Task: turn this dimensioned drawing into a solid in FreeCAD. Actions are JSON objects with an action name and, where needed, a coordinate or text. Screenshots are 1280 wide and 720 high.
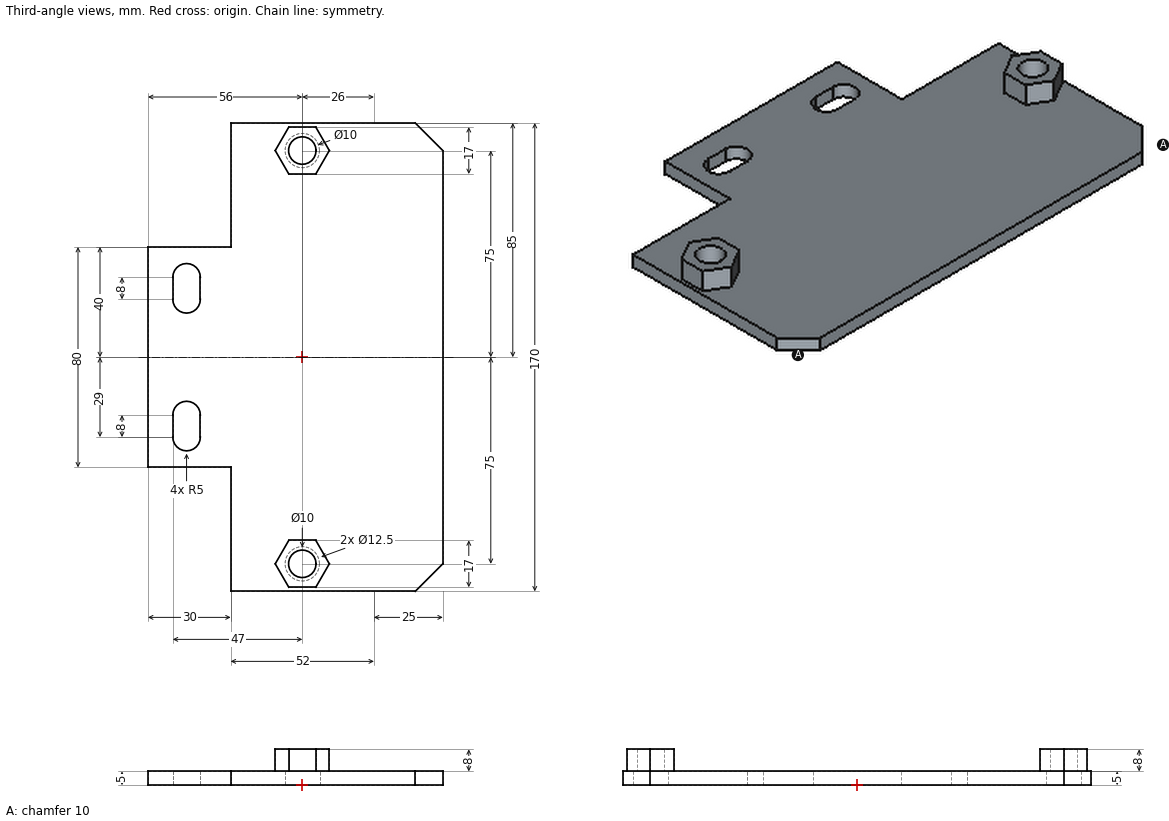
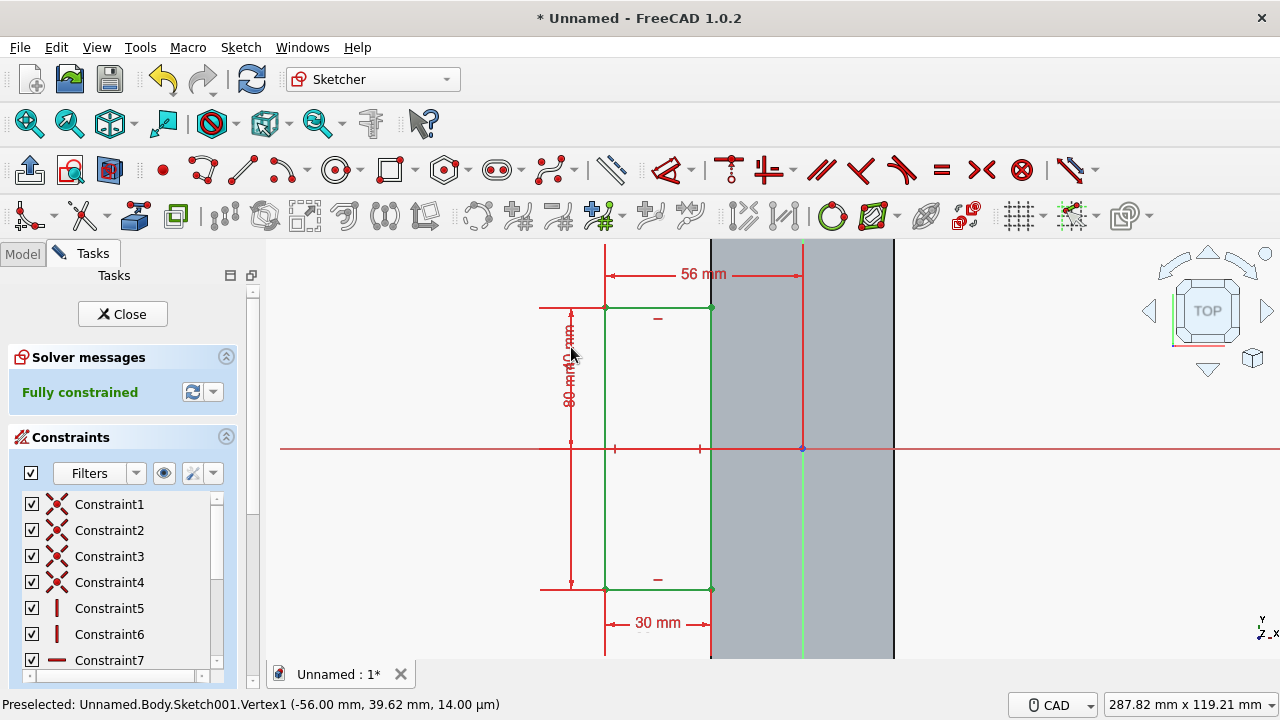
{"action": "left_click", "coordinate": [123, 314]}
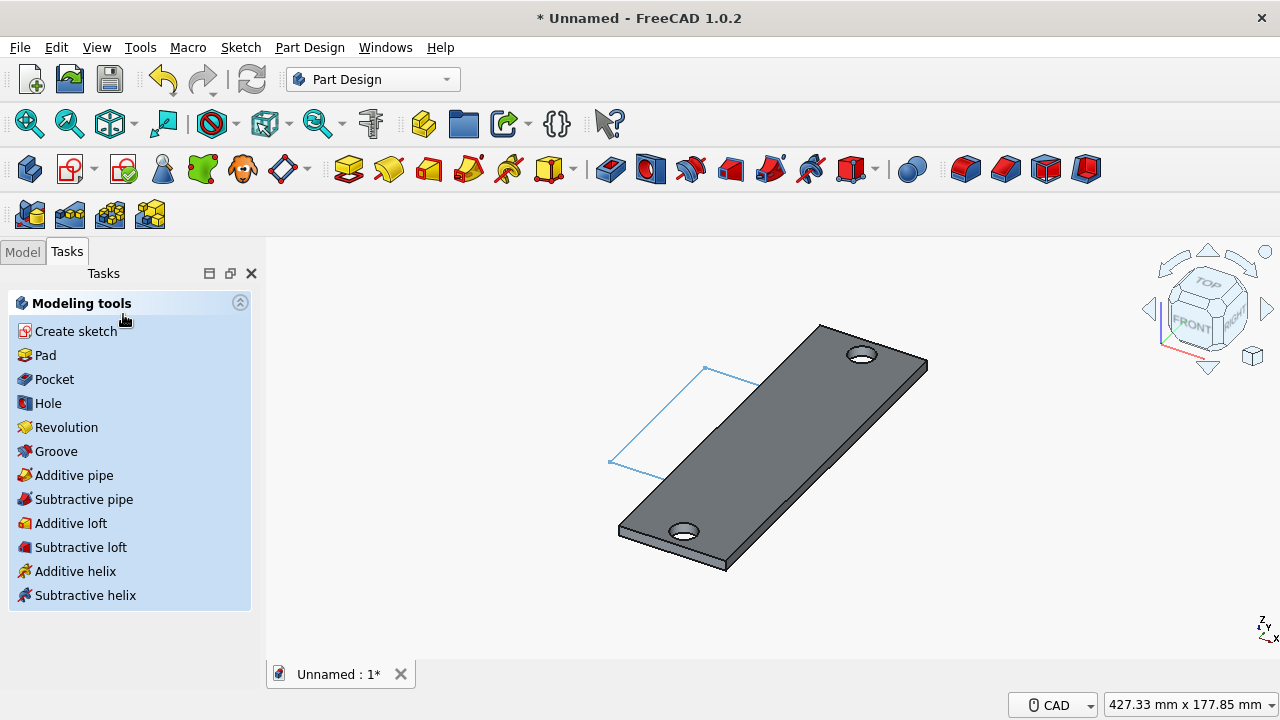
{"action": "left_click", "coordinate": [350, 170]}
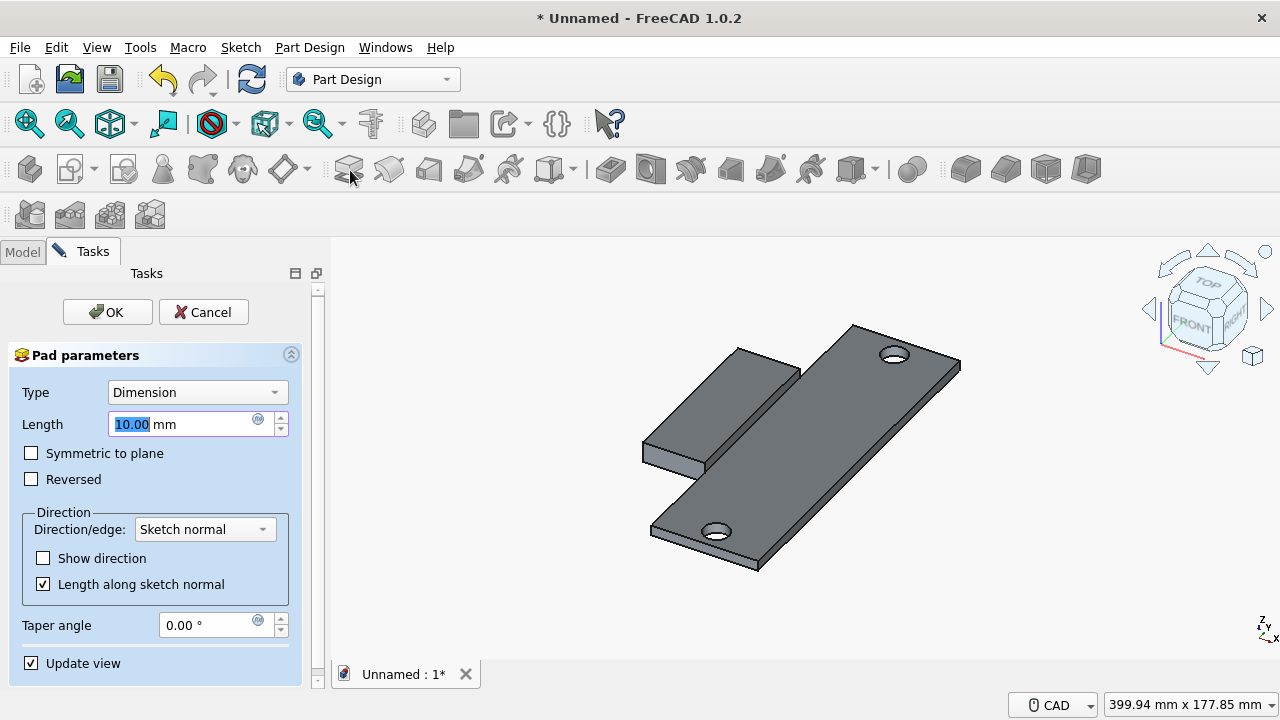
{"action": "type", "text": "5"}
{"action": "key", "text": "Tab"}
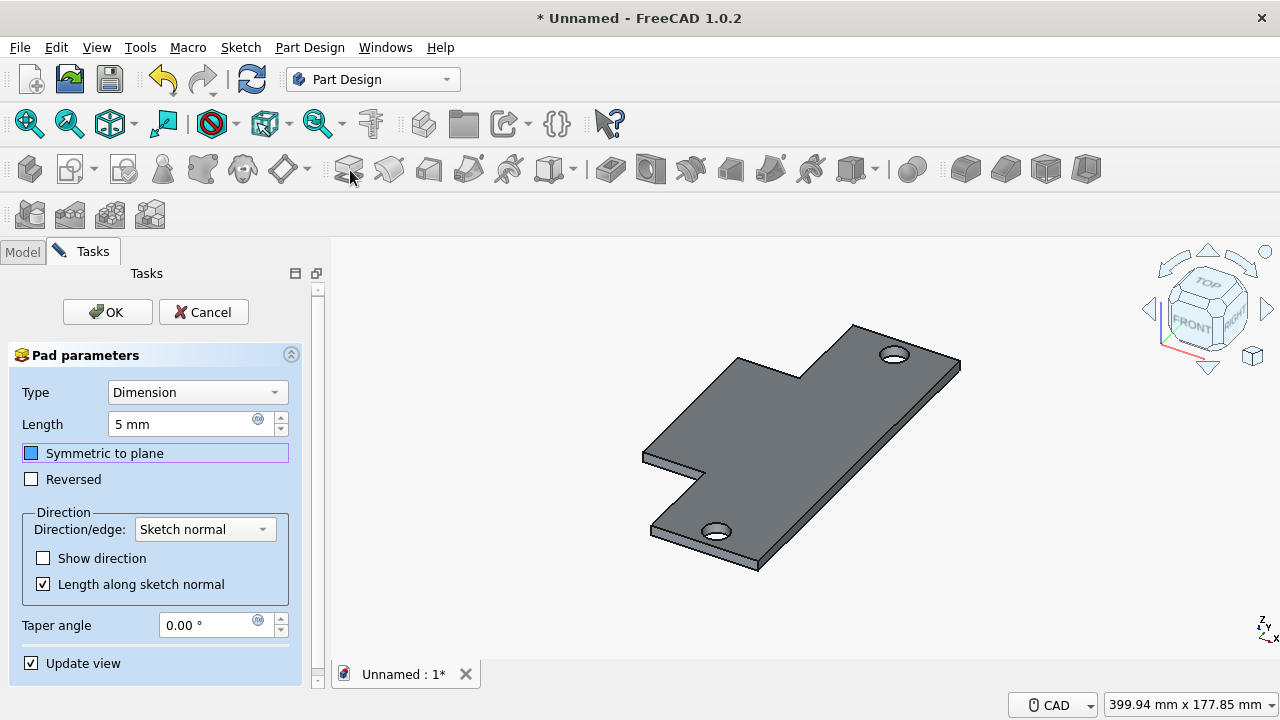
{"action": "left_click", "coordinate": [108, 312]}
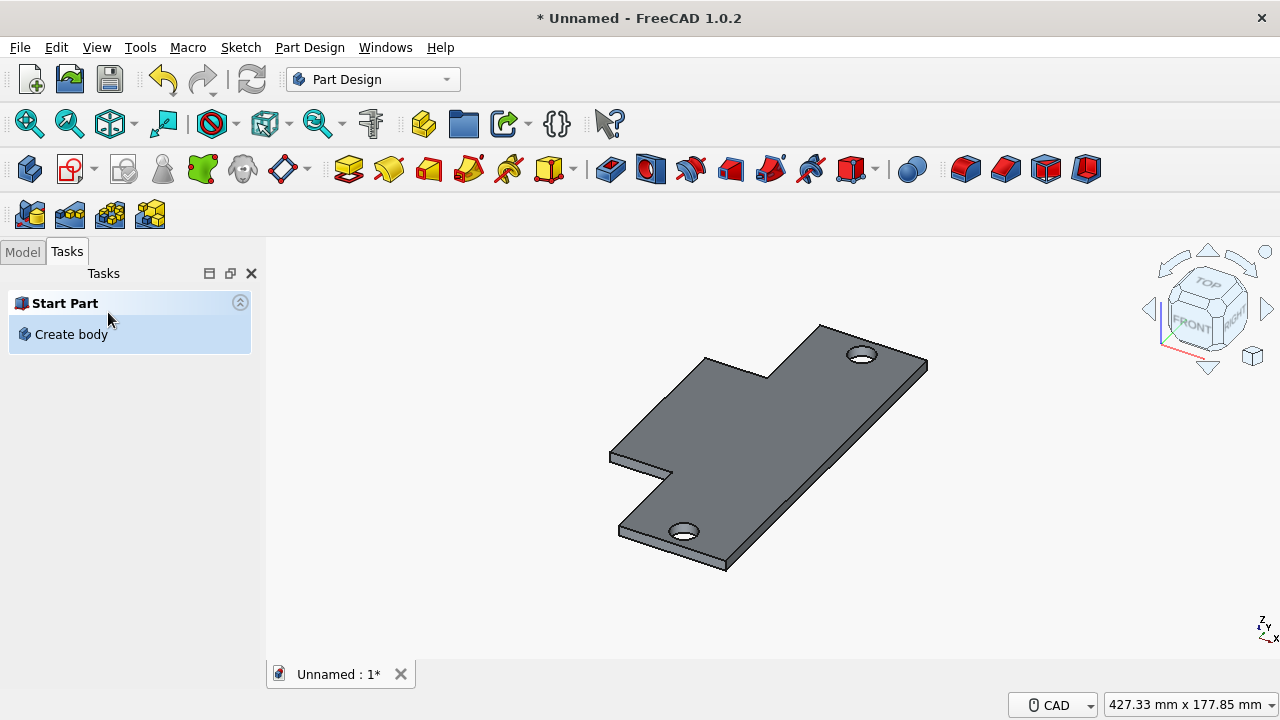
{"action": "left_click", "coordinate": [742, 432]}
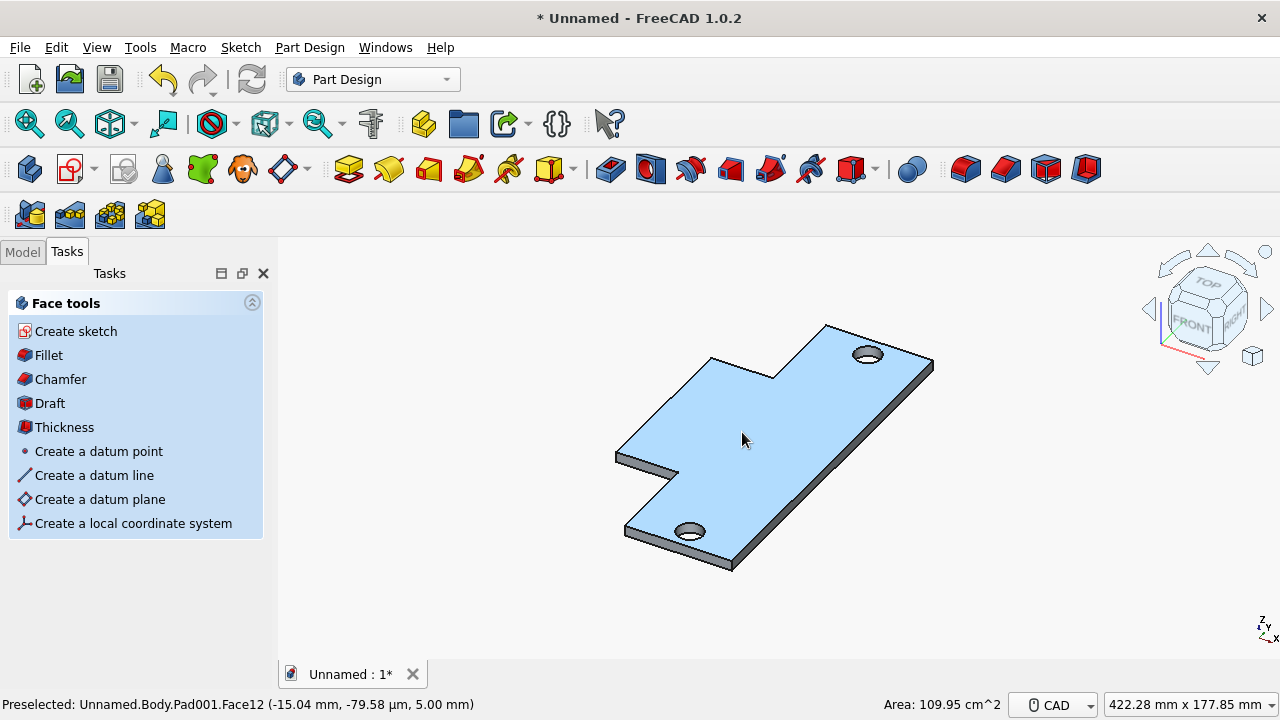
{"action": "left_click", "coordinate": [70, 170]}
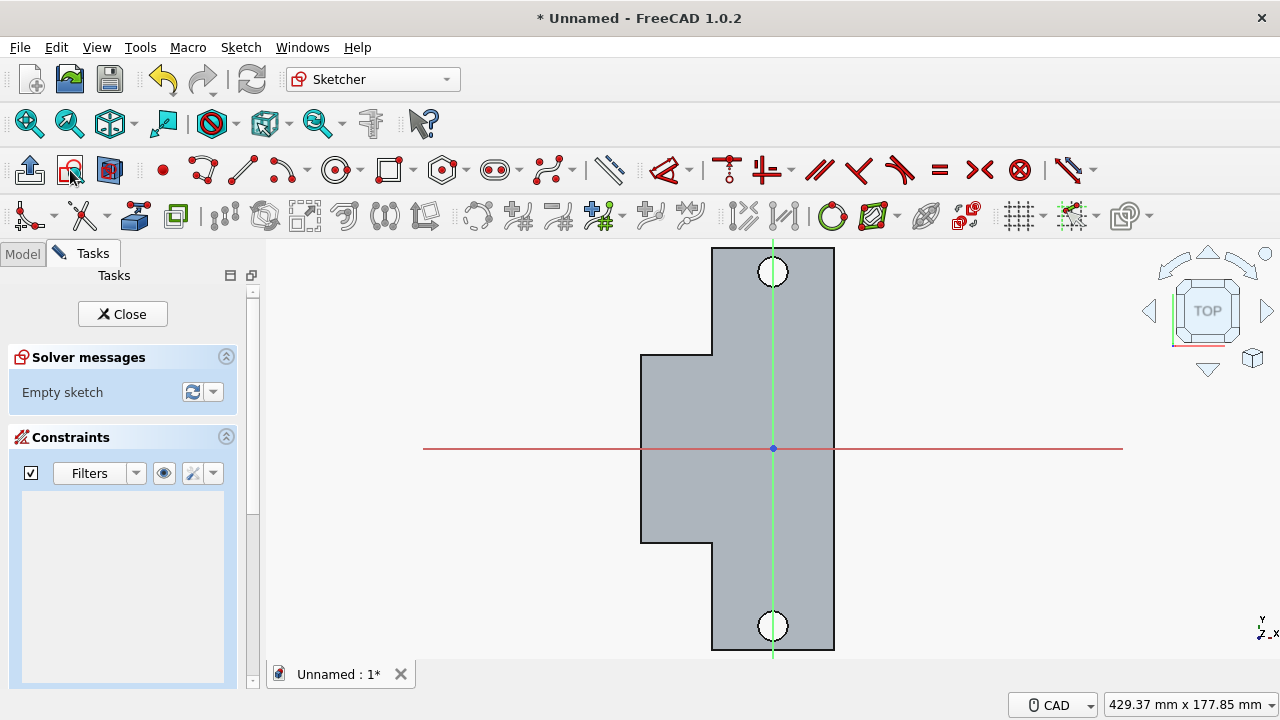
{"action": "scroll", "coordinate": [744, 449], "scroll_direction": "up", "scroll_amount": 2}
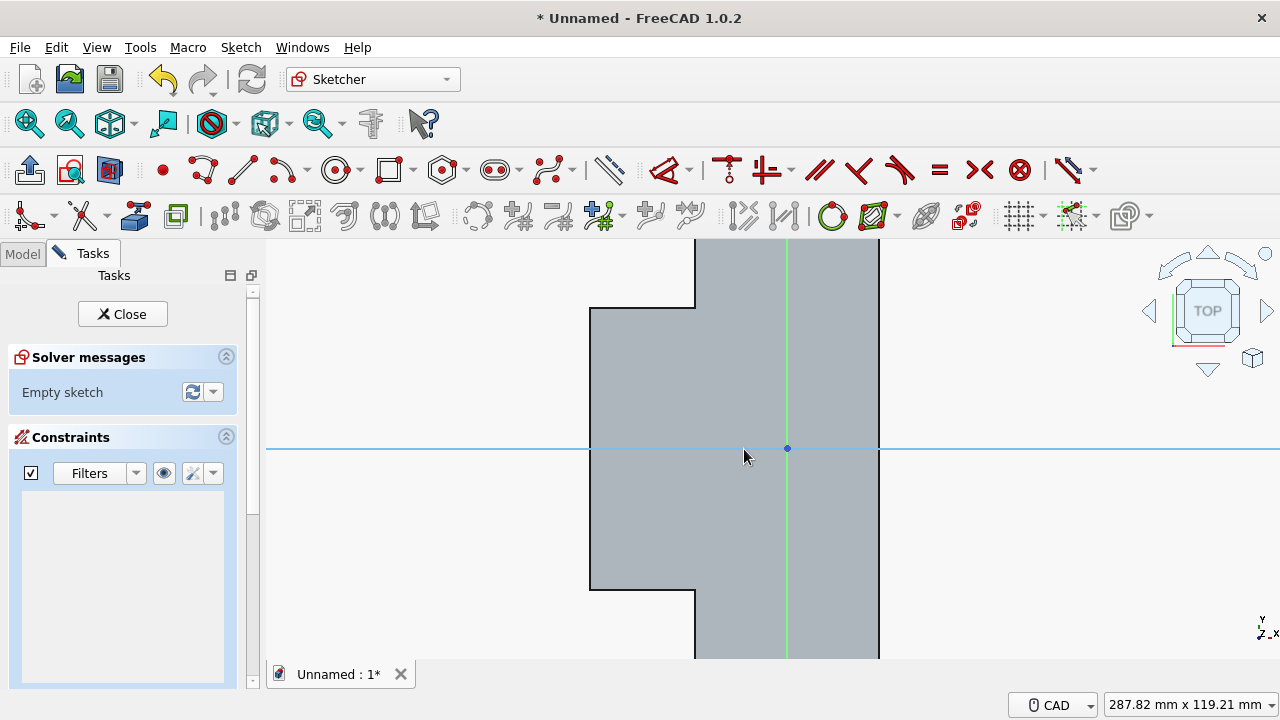
{"action": "left_click", "coordinate": [496, 170]}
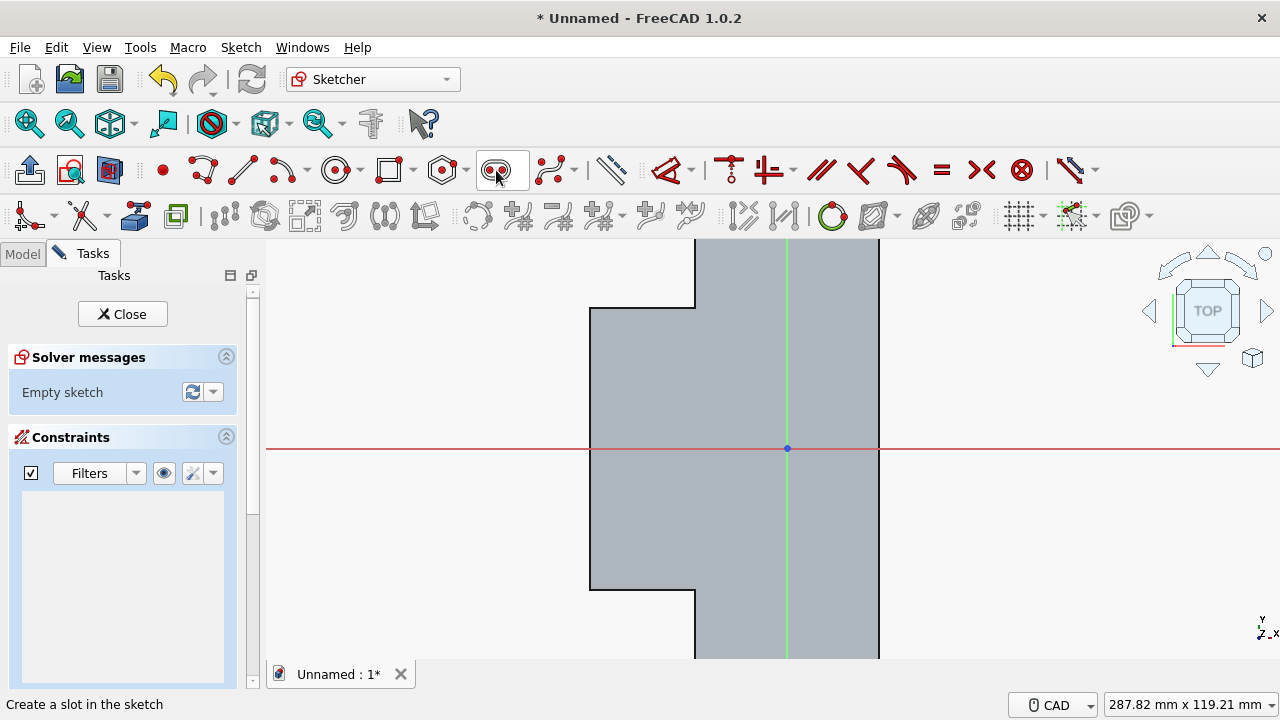
{"action": "scroll", "coordinate": [639, 551], "scroll_direction": "up", "scroll_amount": 2}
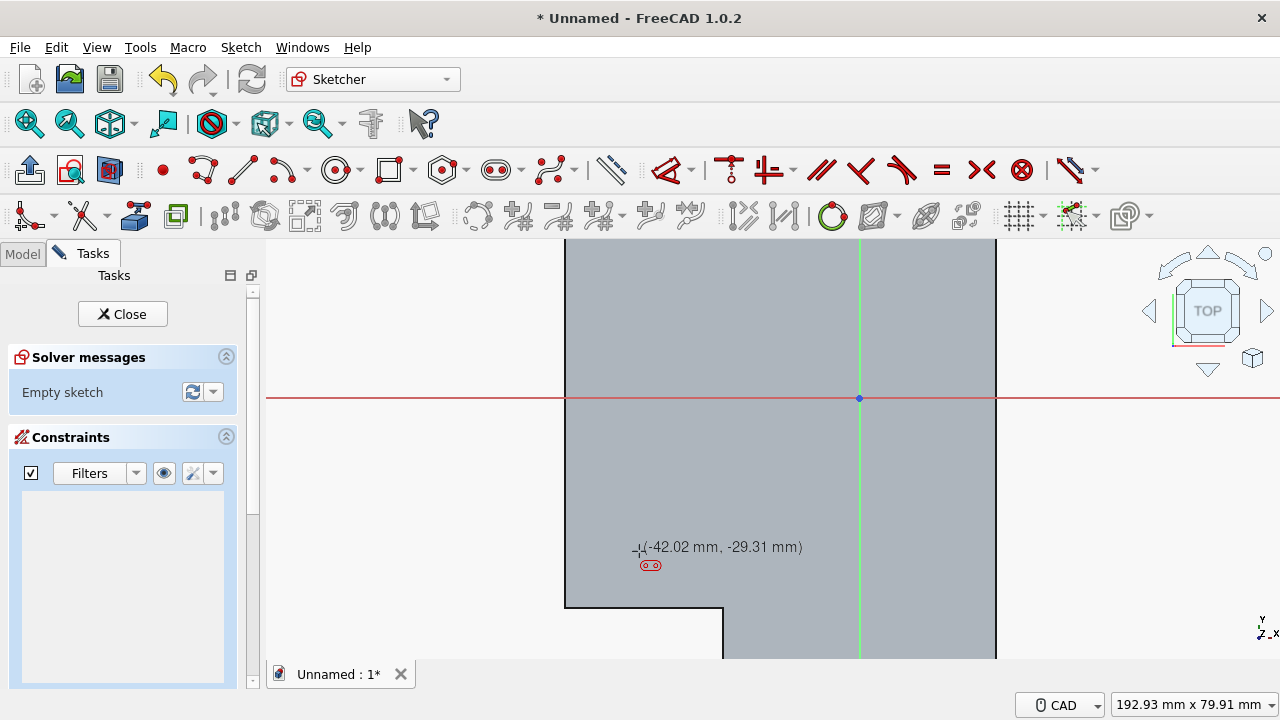
{"action": "left_click", "coordinate": [639, 551]}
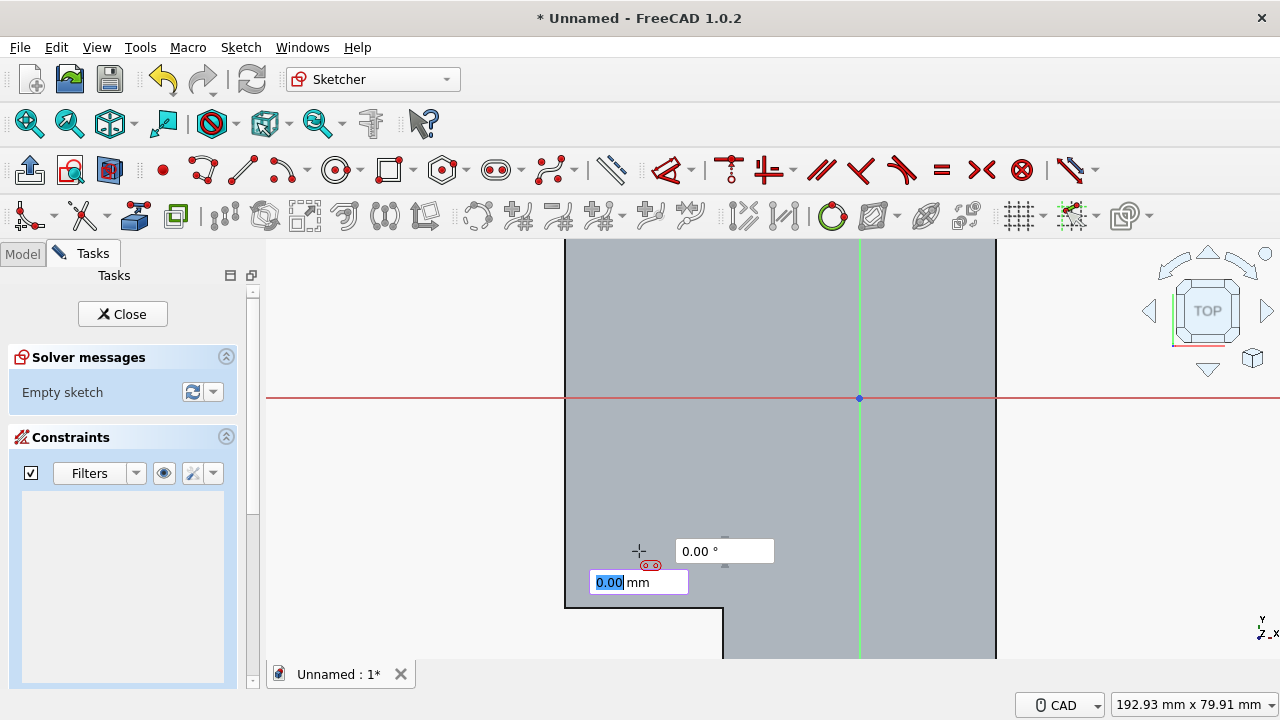
{"action": "left_click", "coordinate": [639, 508]}